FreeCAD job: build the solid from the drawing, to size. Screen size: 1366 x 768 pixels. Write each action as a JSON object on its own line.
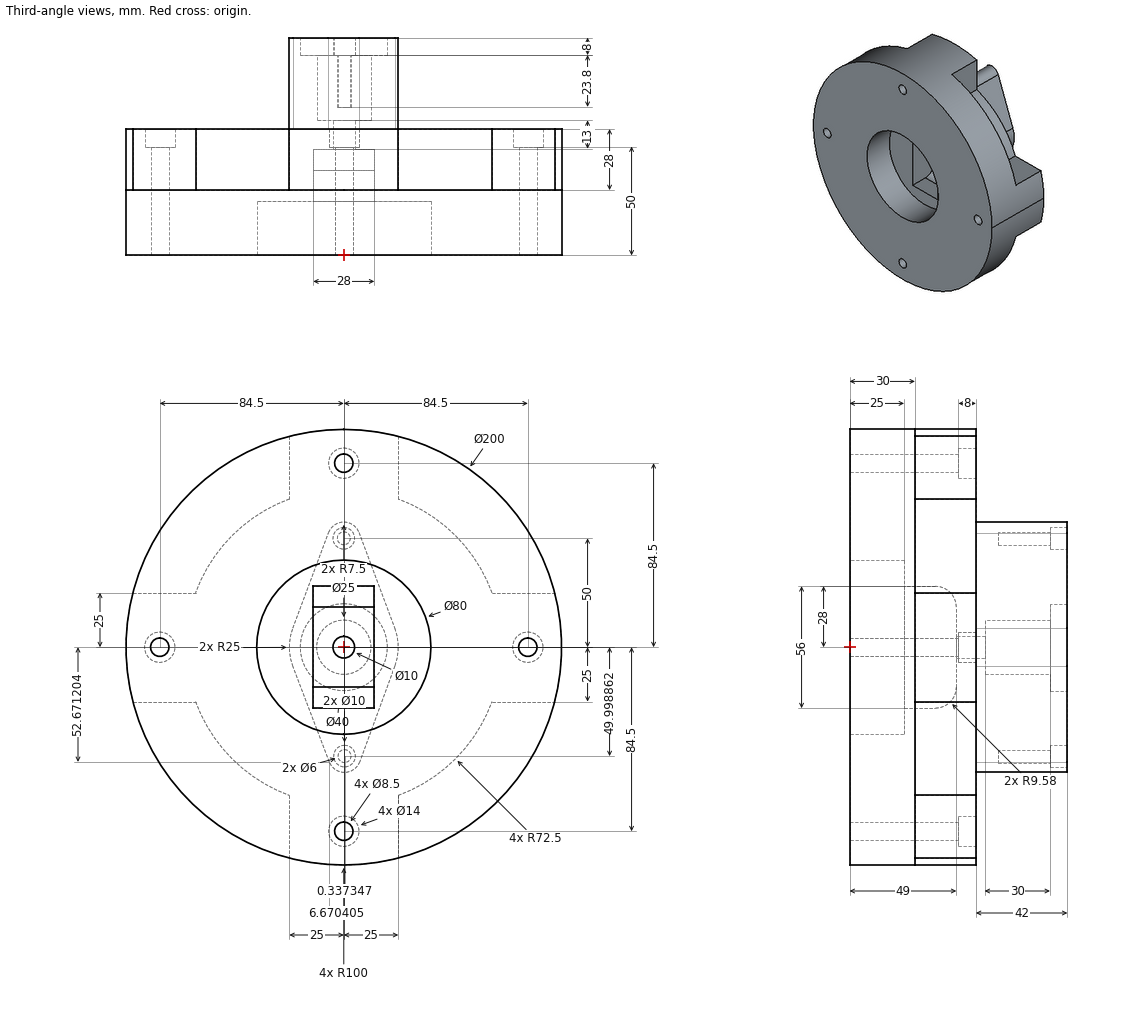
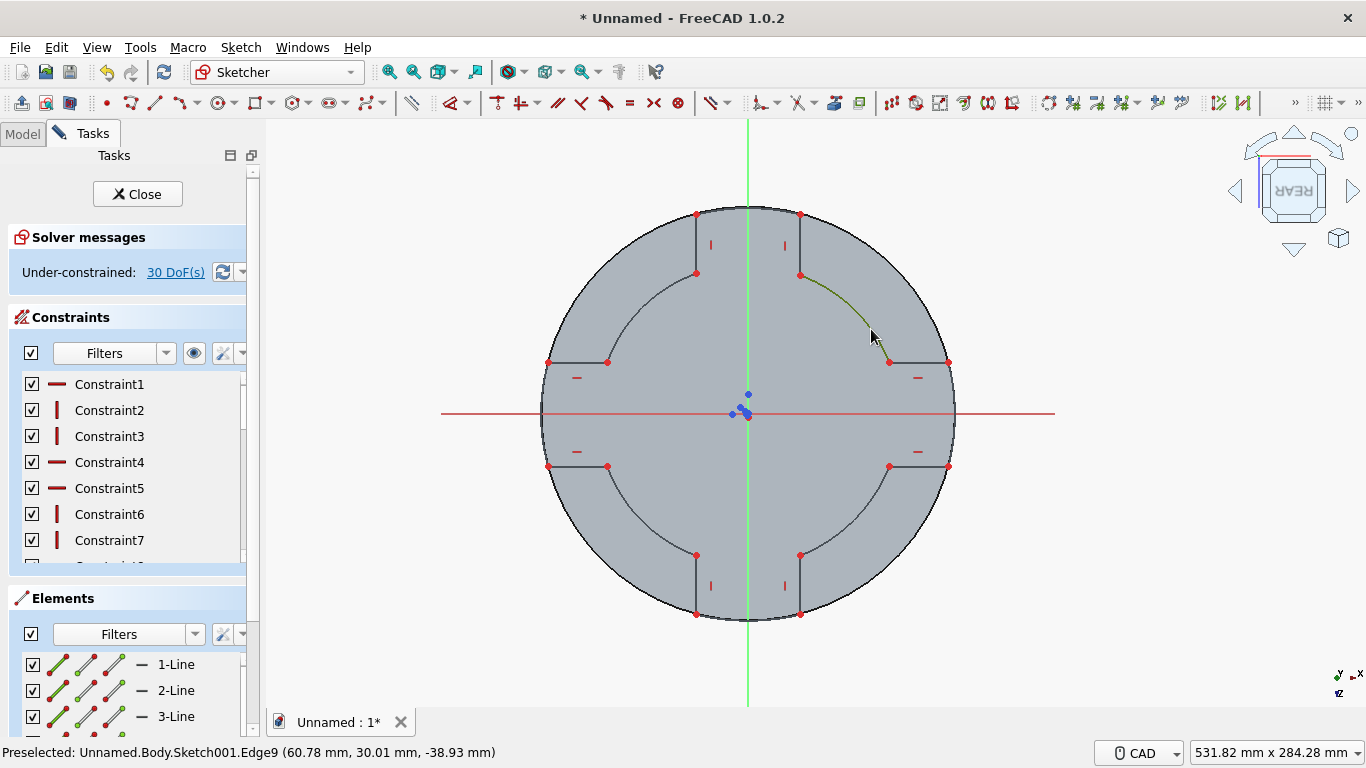
{"action": "left_click", "coordinate": [662, 291]}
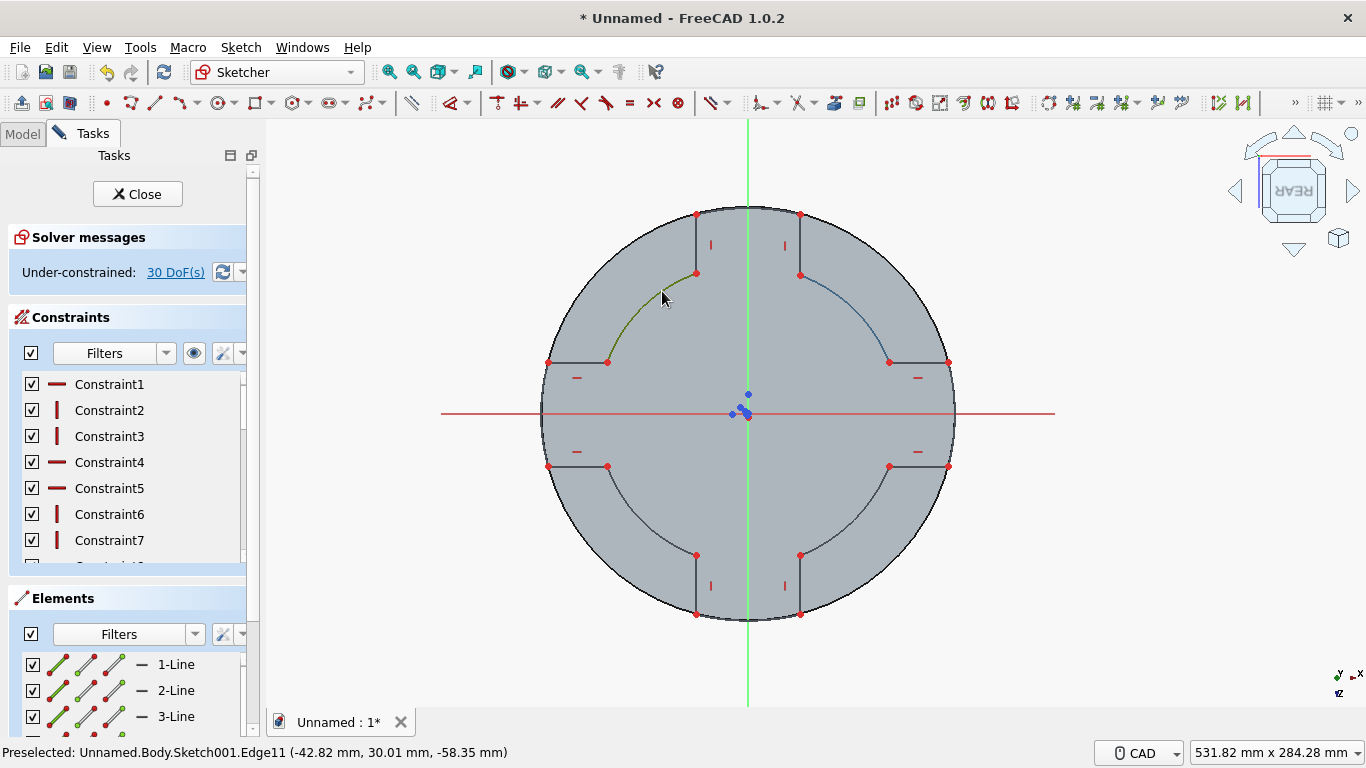
{"action": "key", "text": "c"}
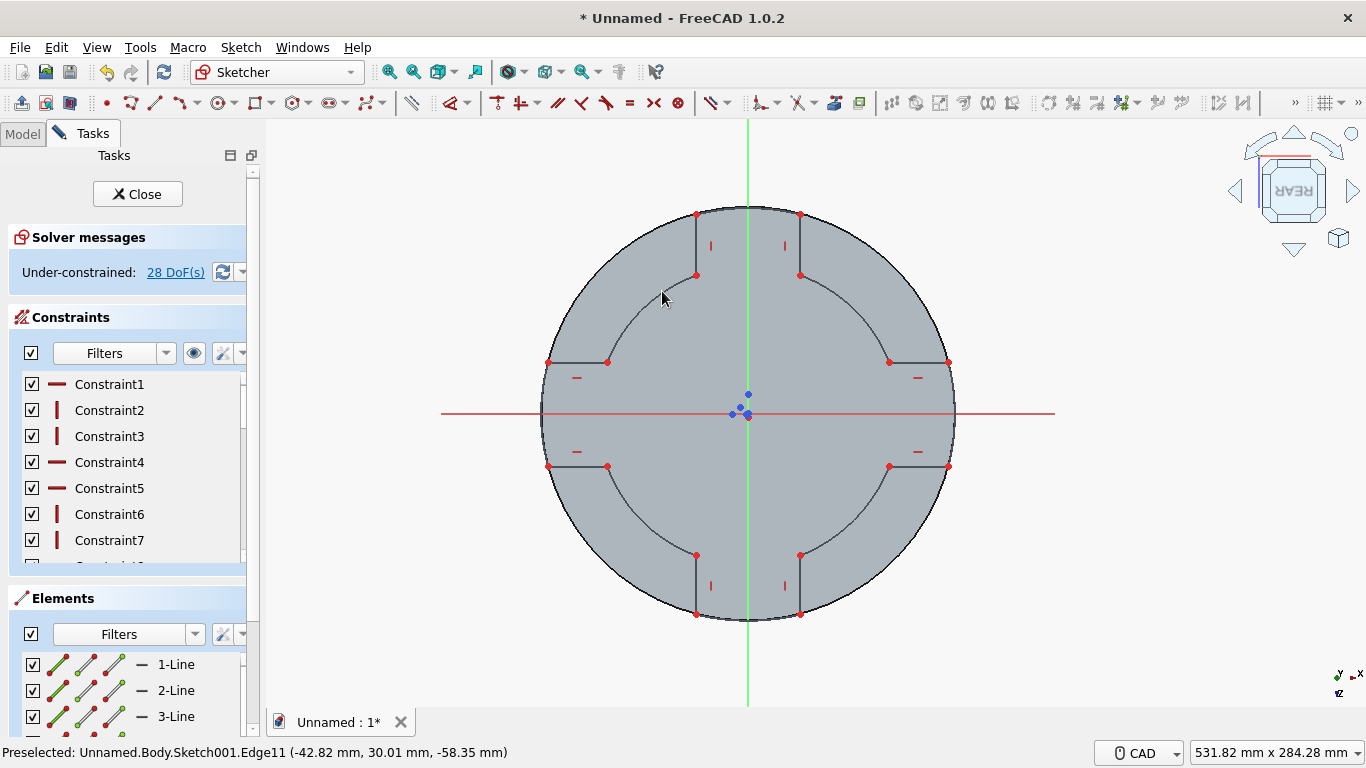
{"action": "left_click", "coordinate": [871, 329]}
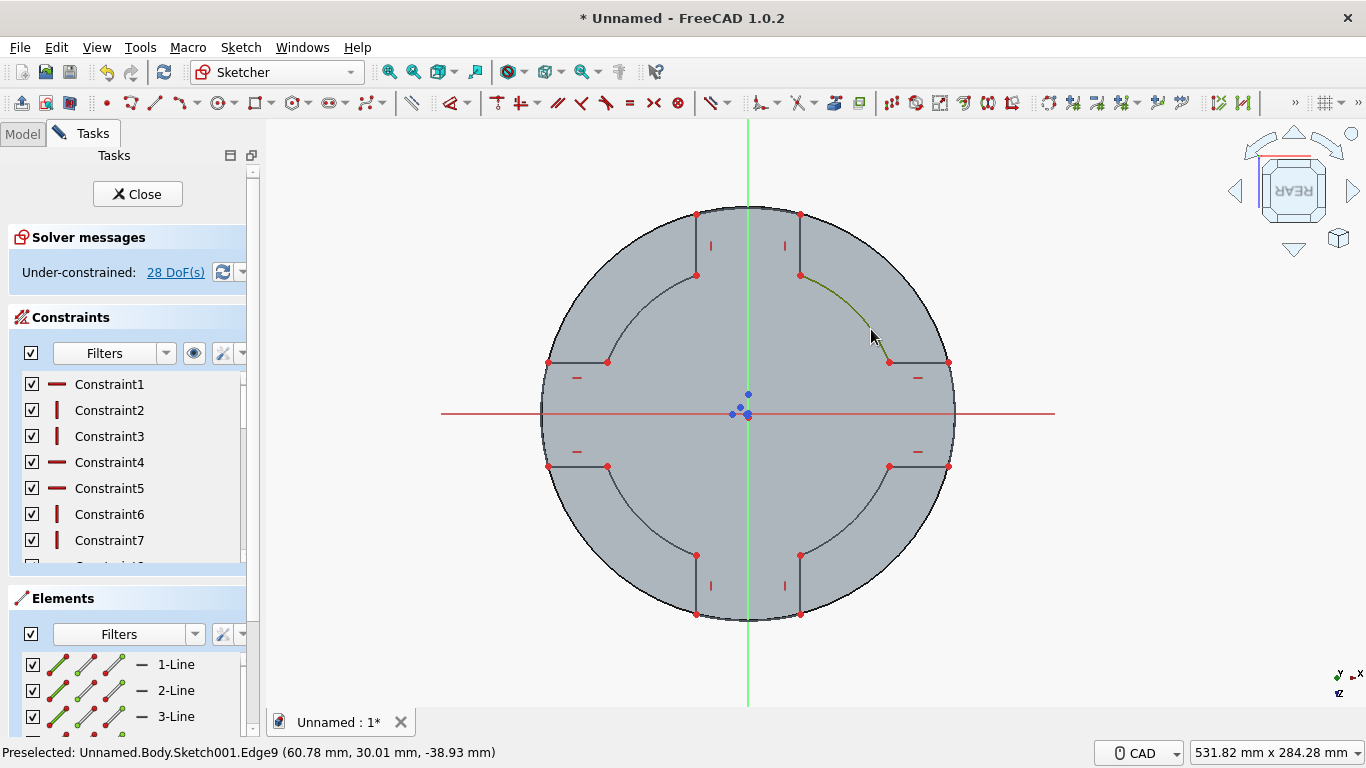
{"action": "left_click", "coordinate": [542, 394]}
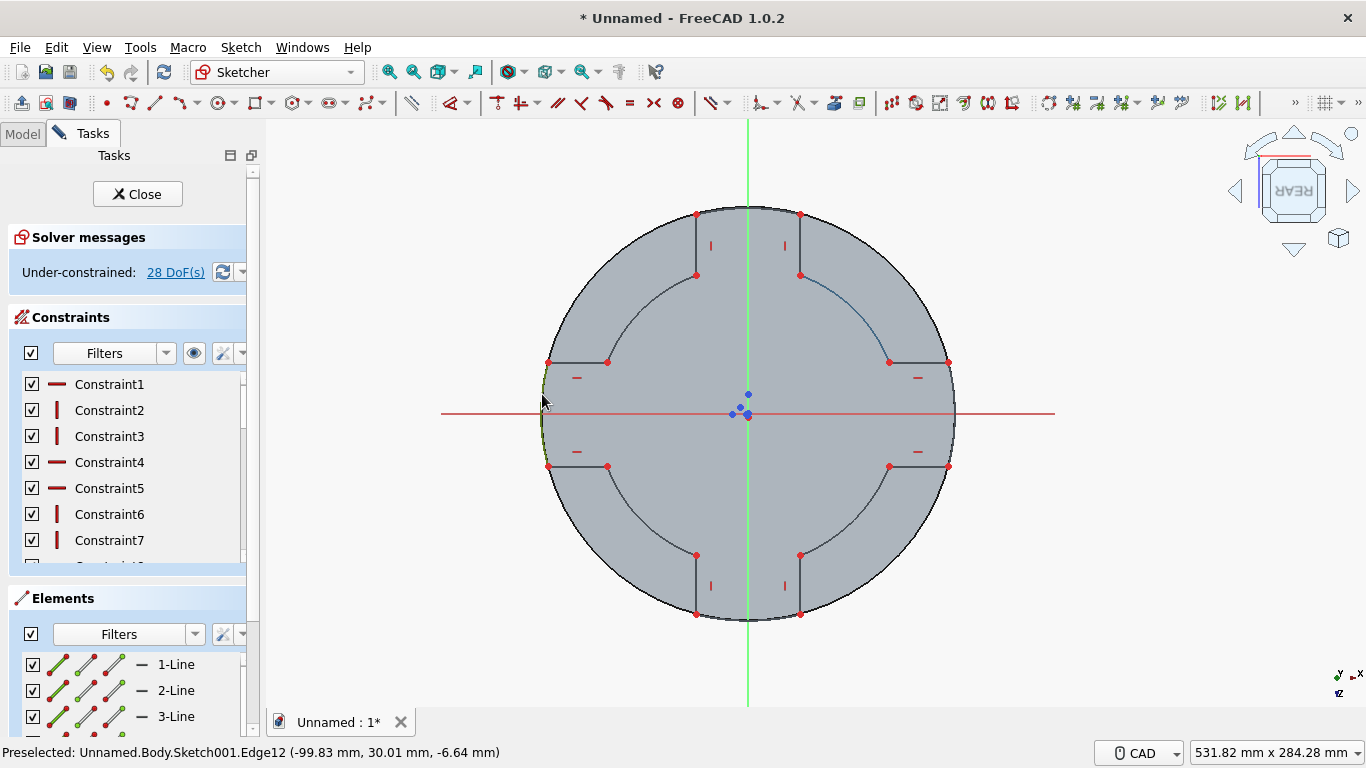
{"action": "key", "text": "c"}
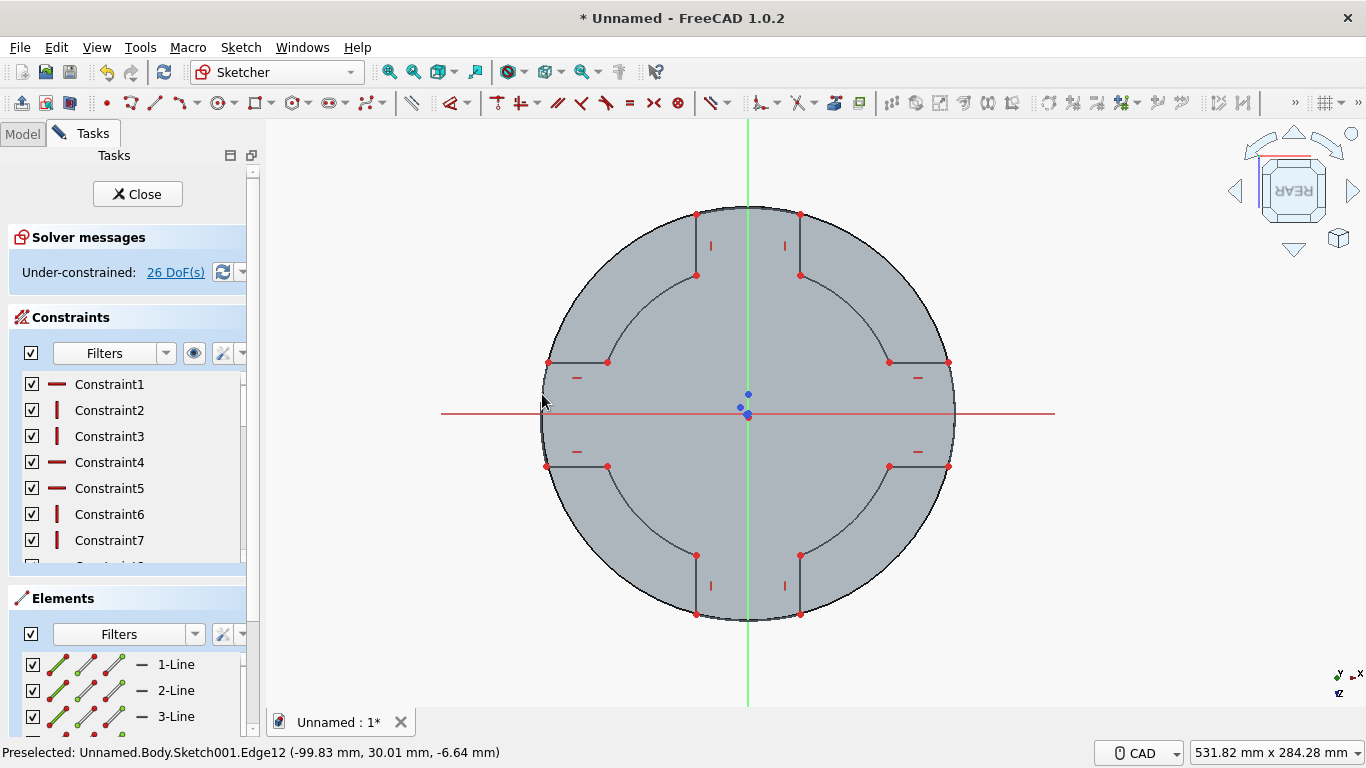
{"action": "left_click", "coordinate": [871, 329]}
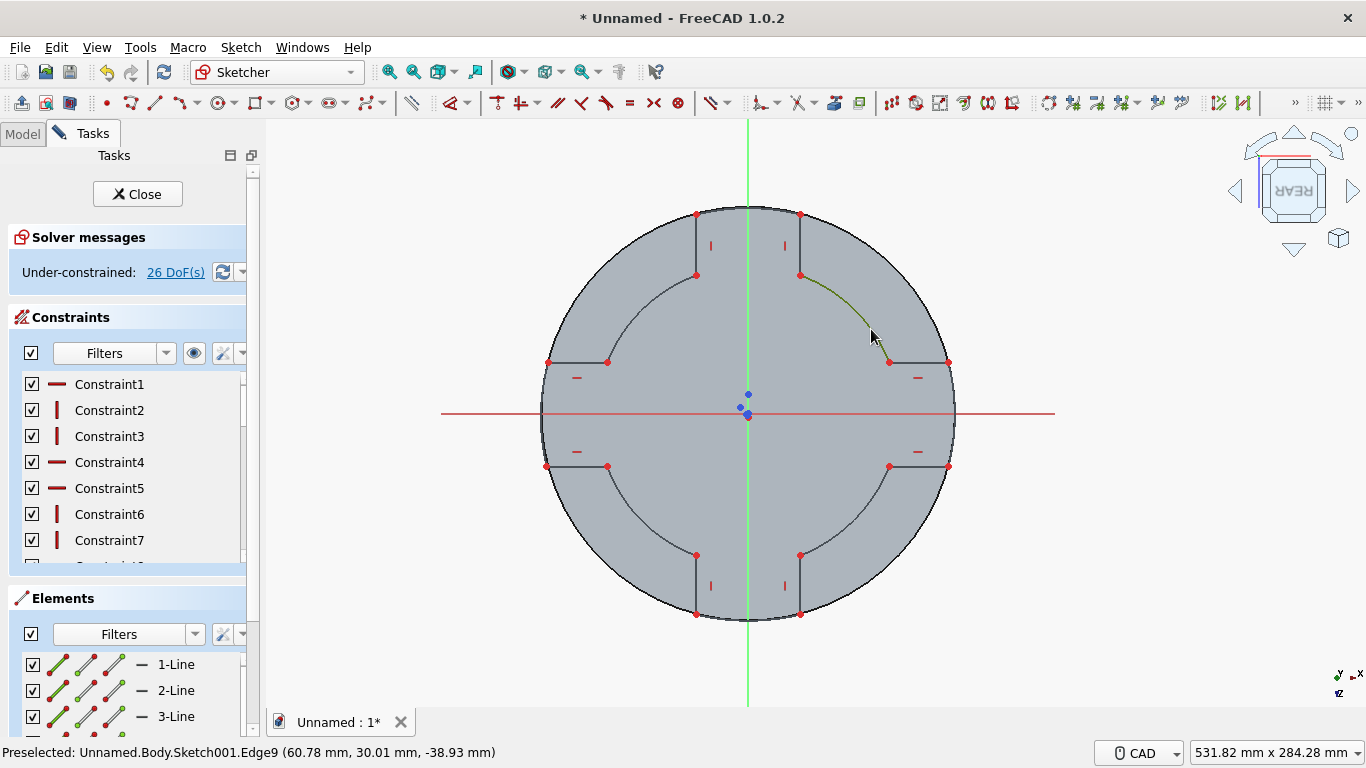
{"action": "left_click", "coordinate": [625, 501]}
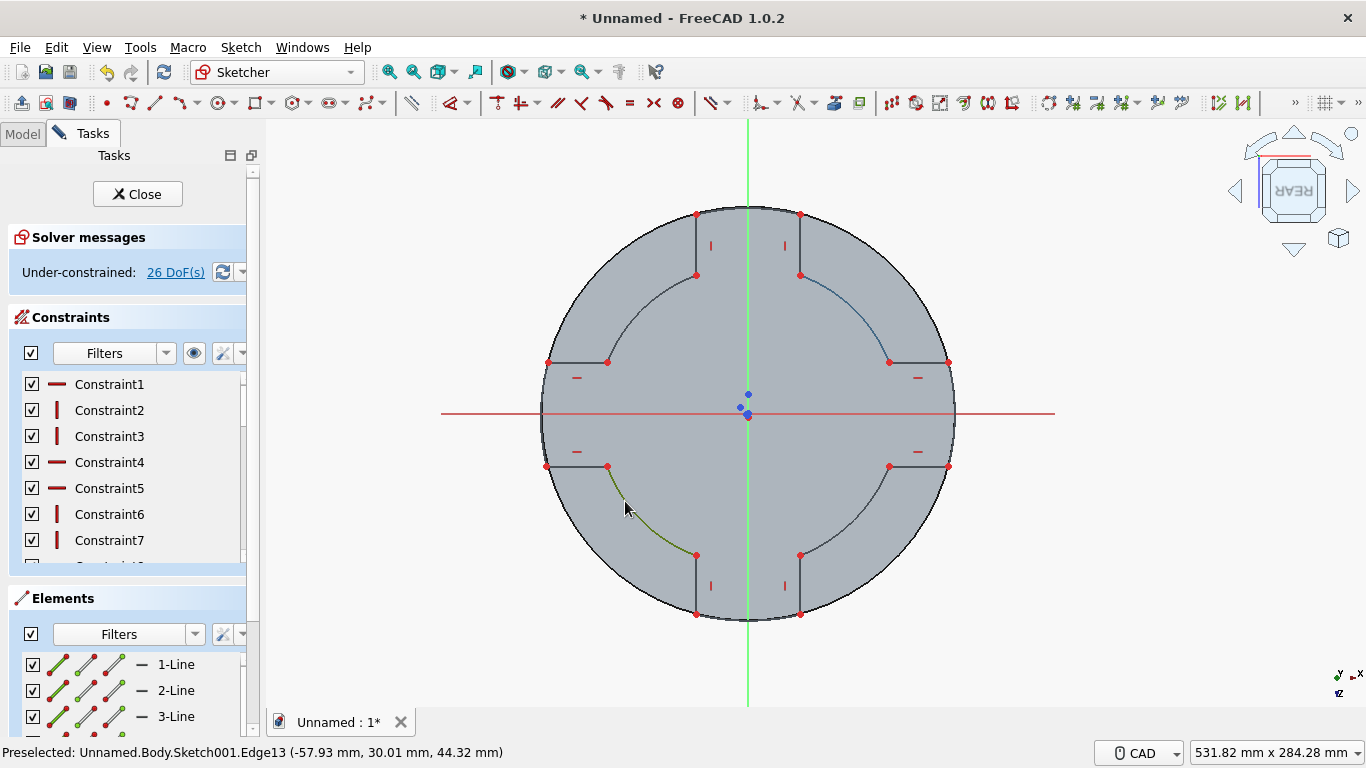
{"action": "key", "text": "c"}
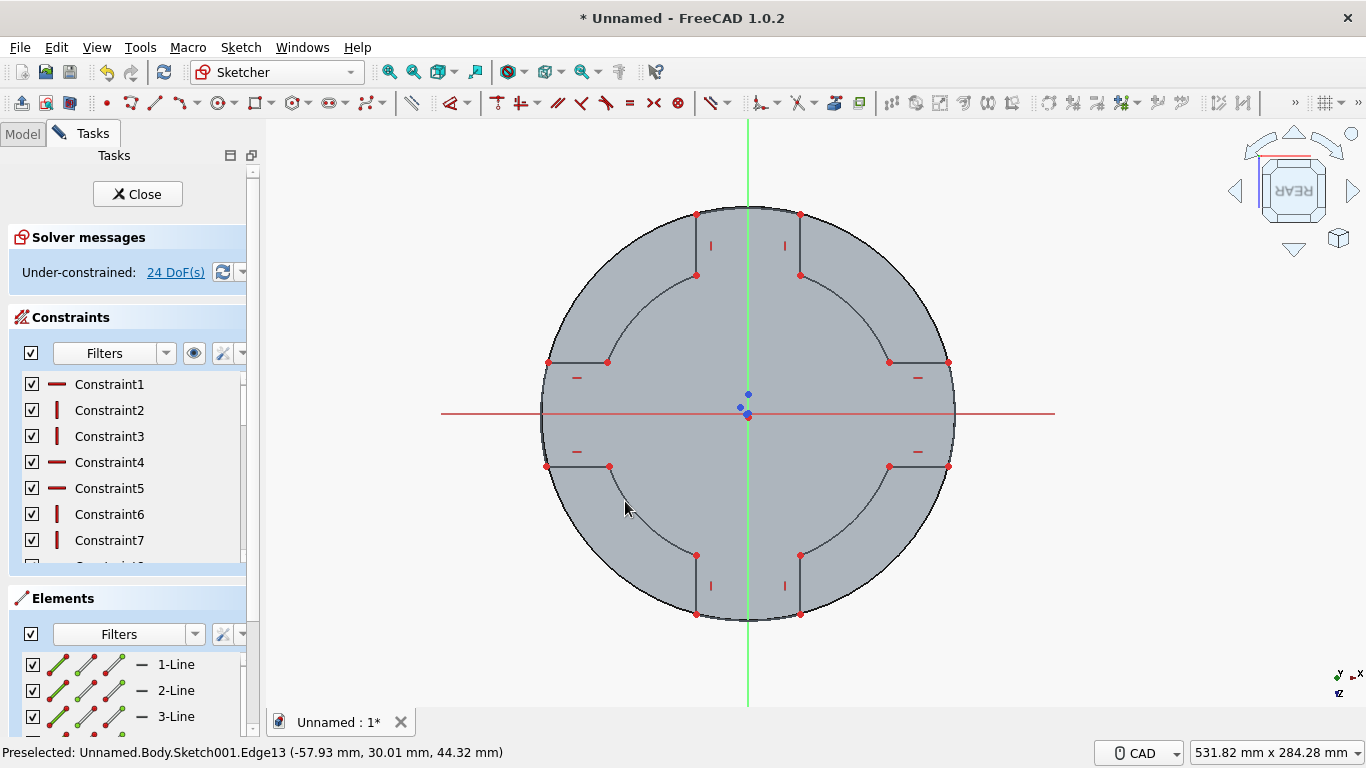
{"action": "left_click", "coordinate": [871, 329]}